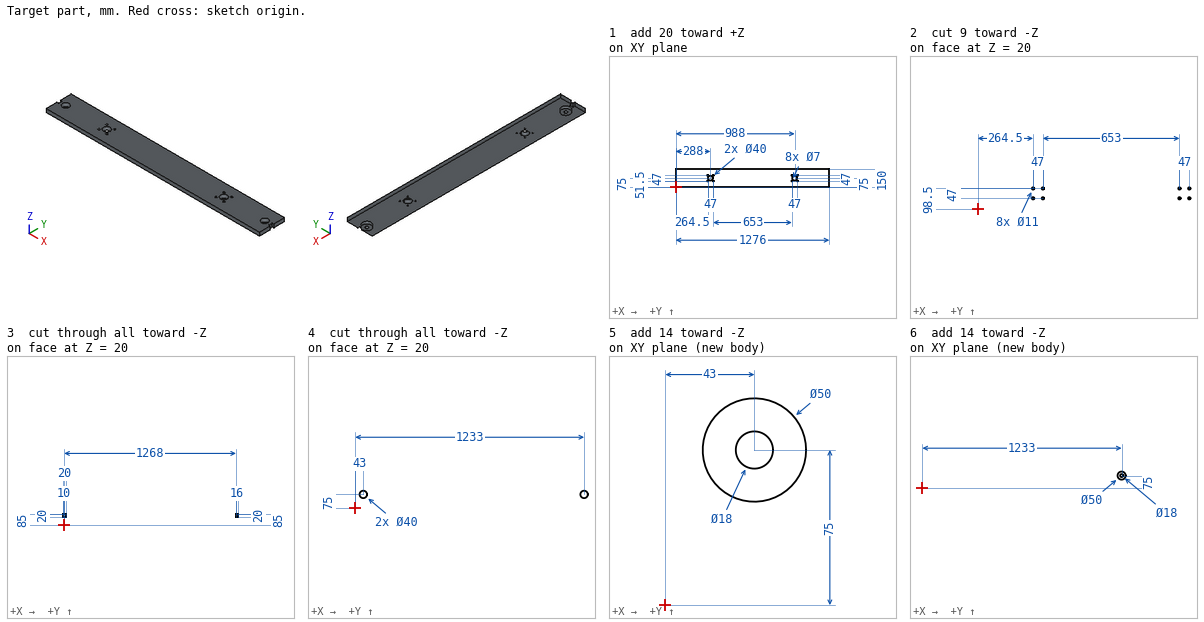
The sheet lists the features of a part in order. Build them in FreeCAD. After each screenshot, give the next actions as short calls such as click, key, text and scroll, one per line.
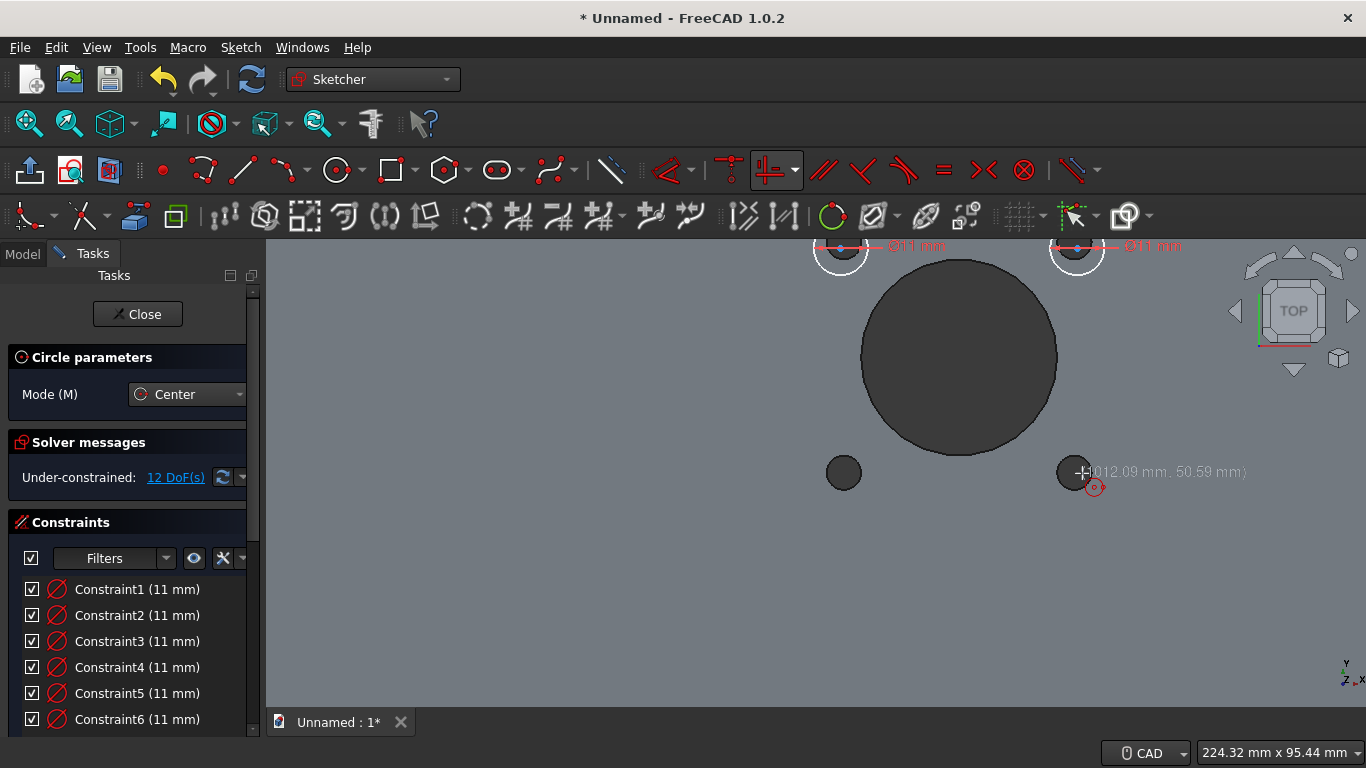
scroll(1082, 473, down, 10)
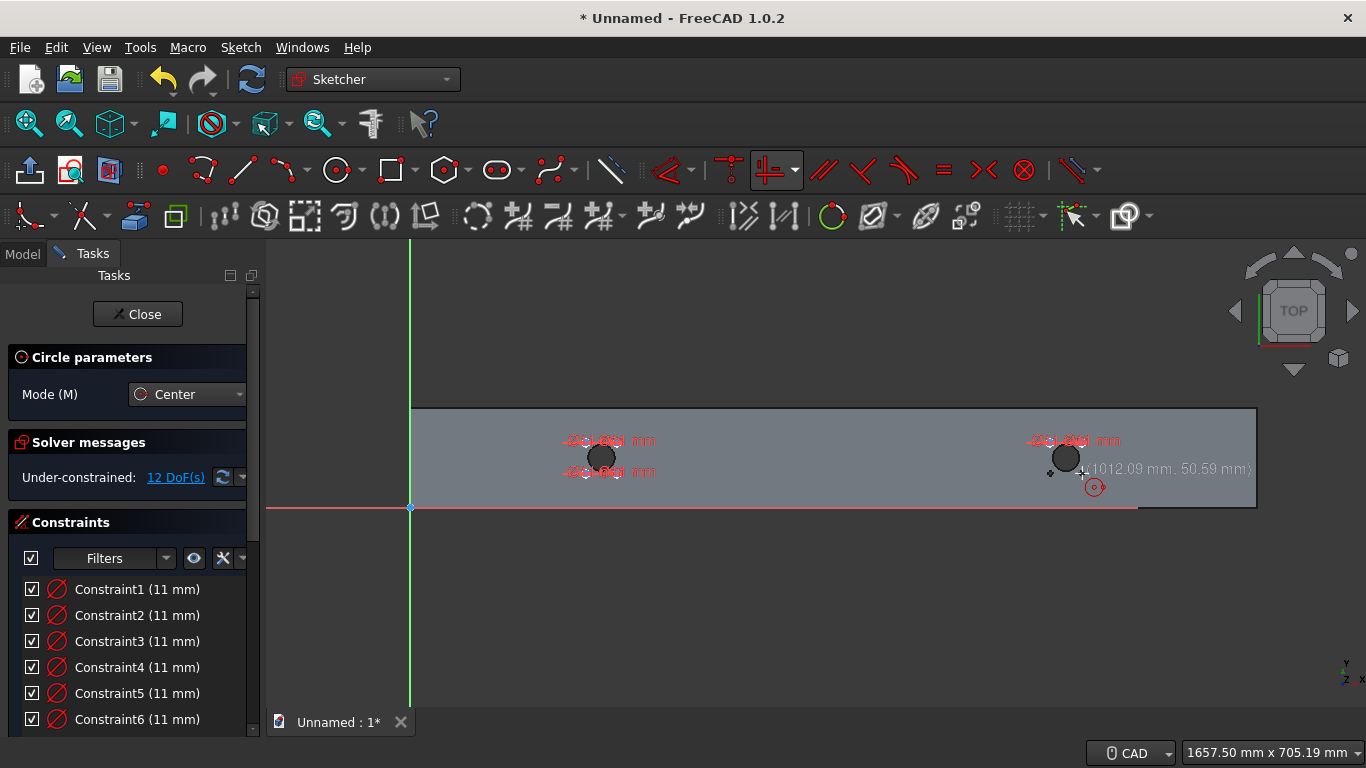
click(1082, 473)
move(1084, 471)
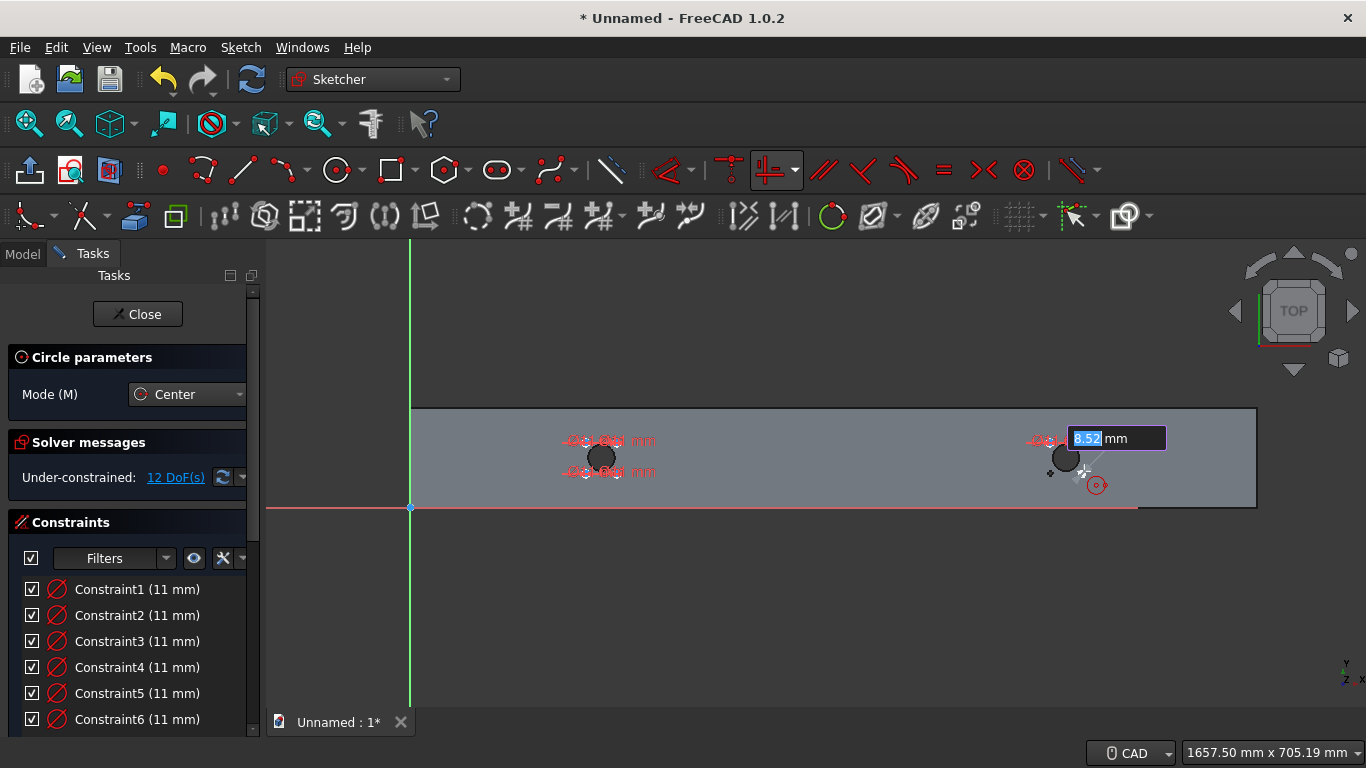
text(11)
key(Return)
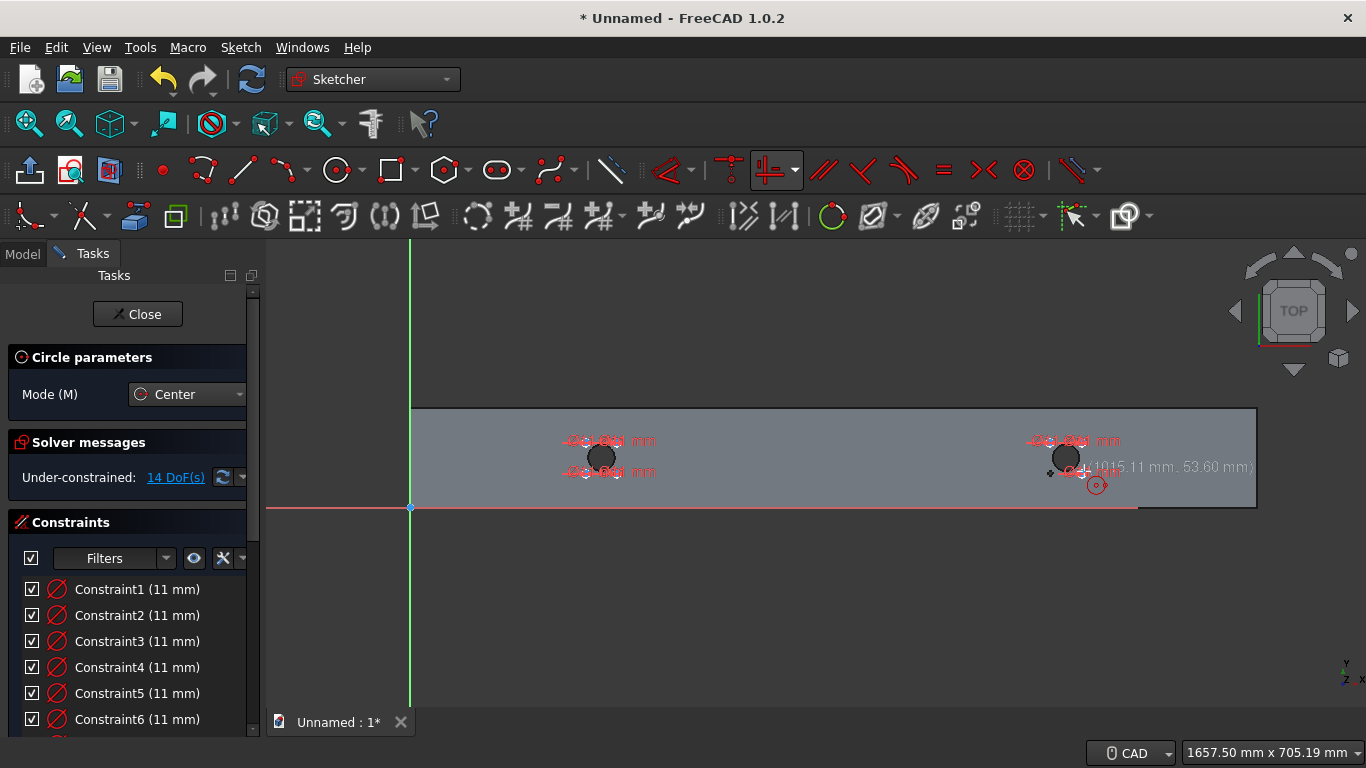
scroll(1050, 473, up, 10)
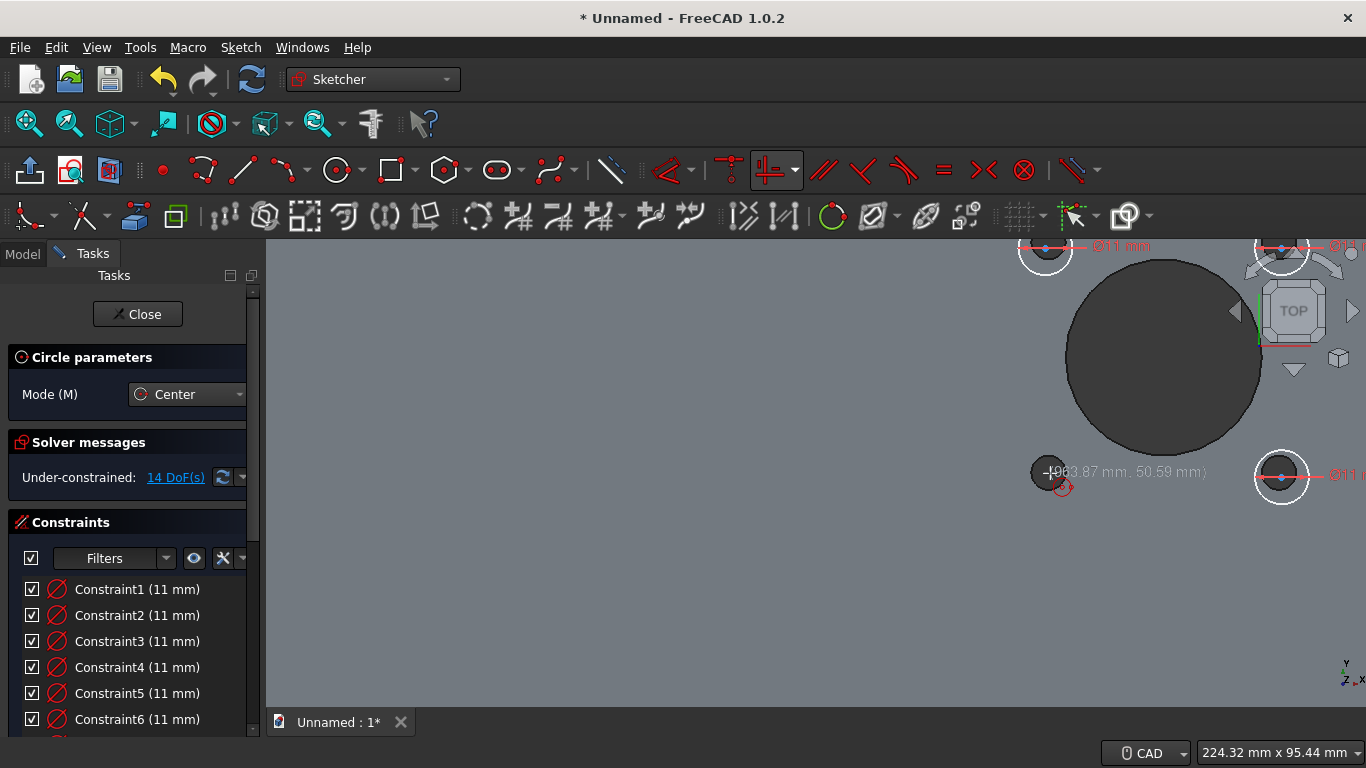
scroll(1050, 473, down, 10)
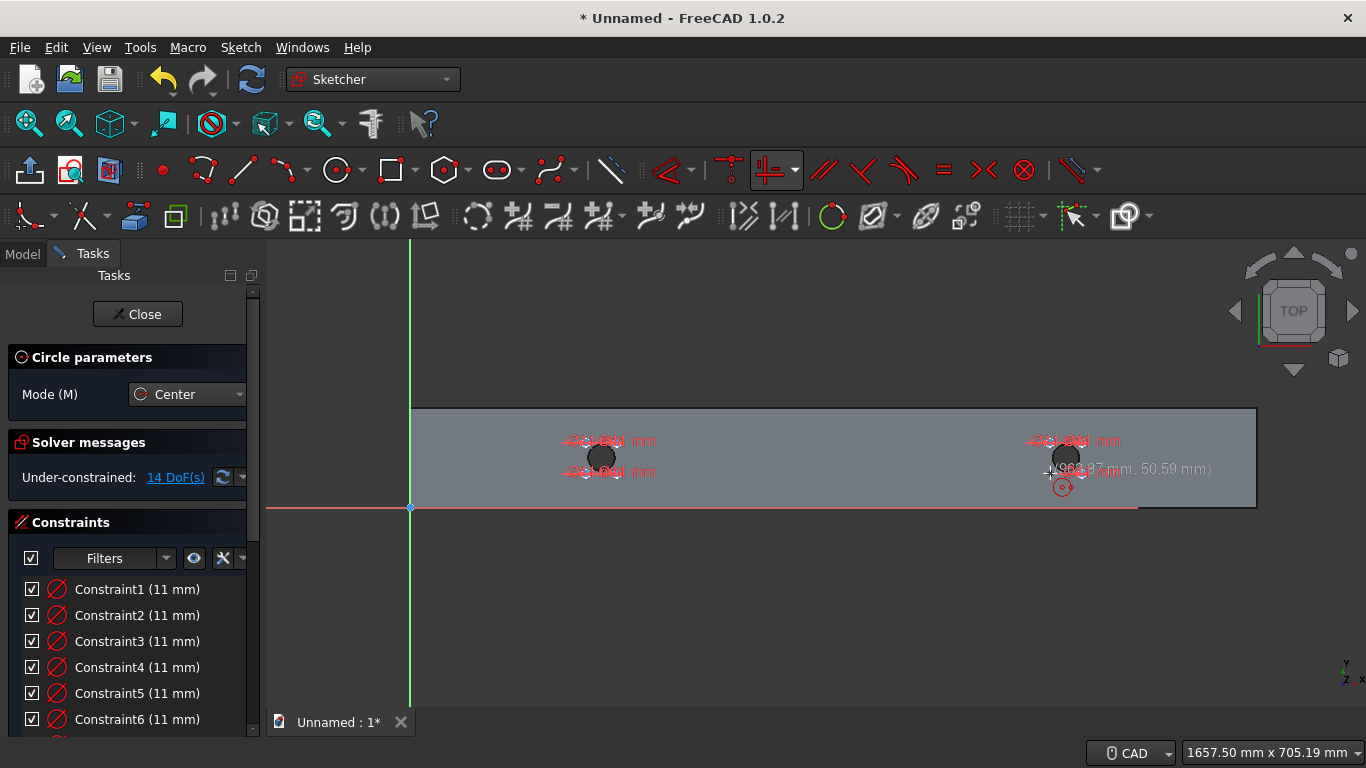
click(1050, 473)
move(1053, 471)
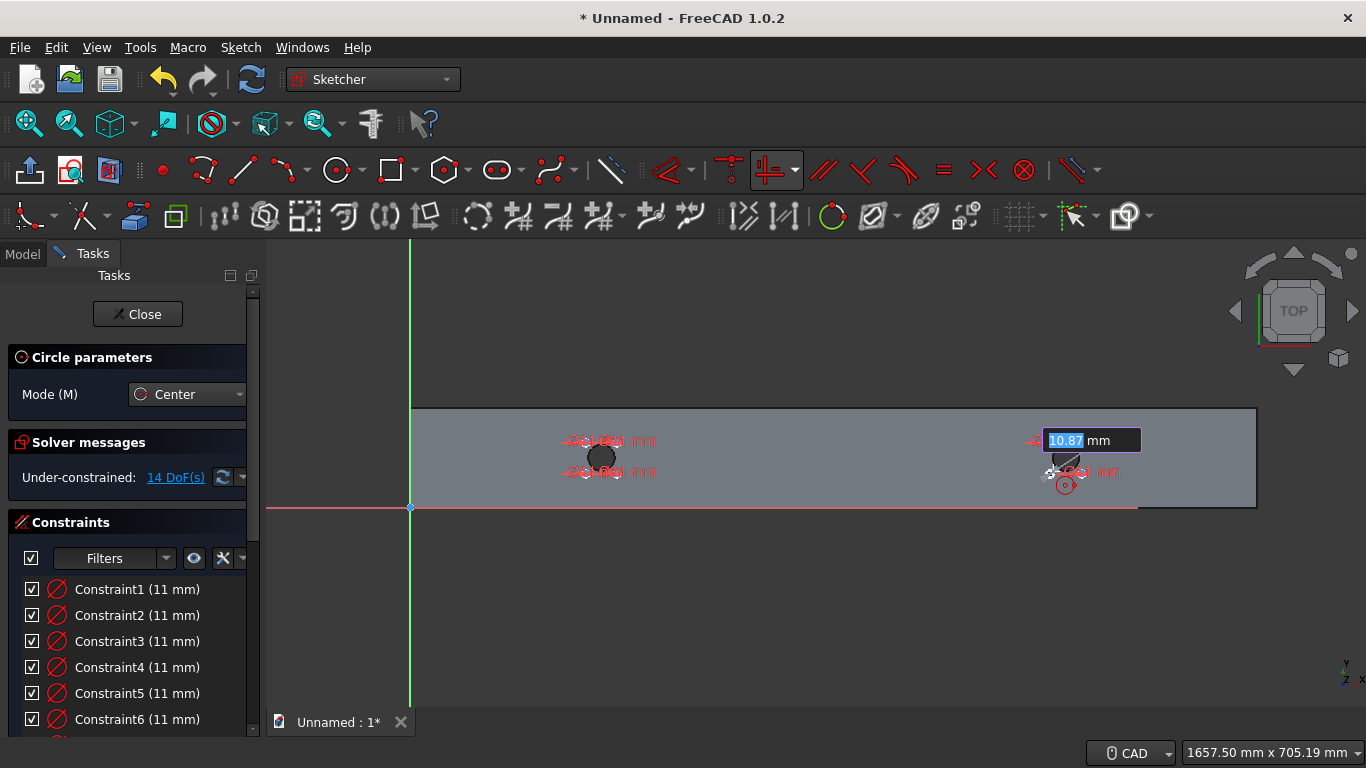
text(11)
key(Return)
key(Escape)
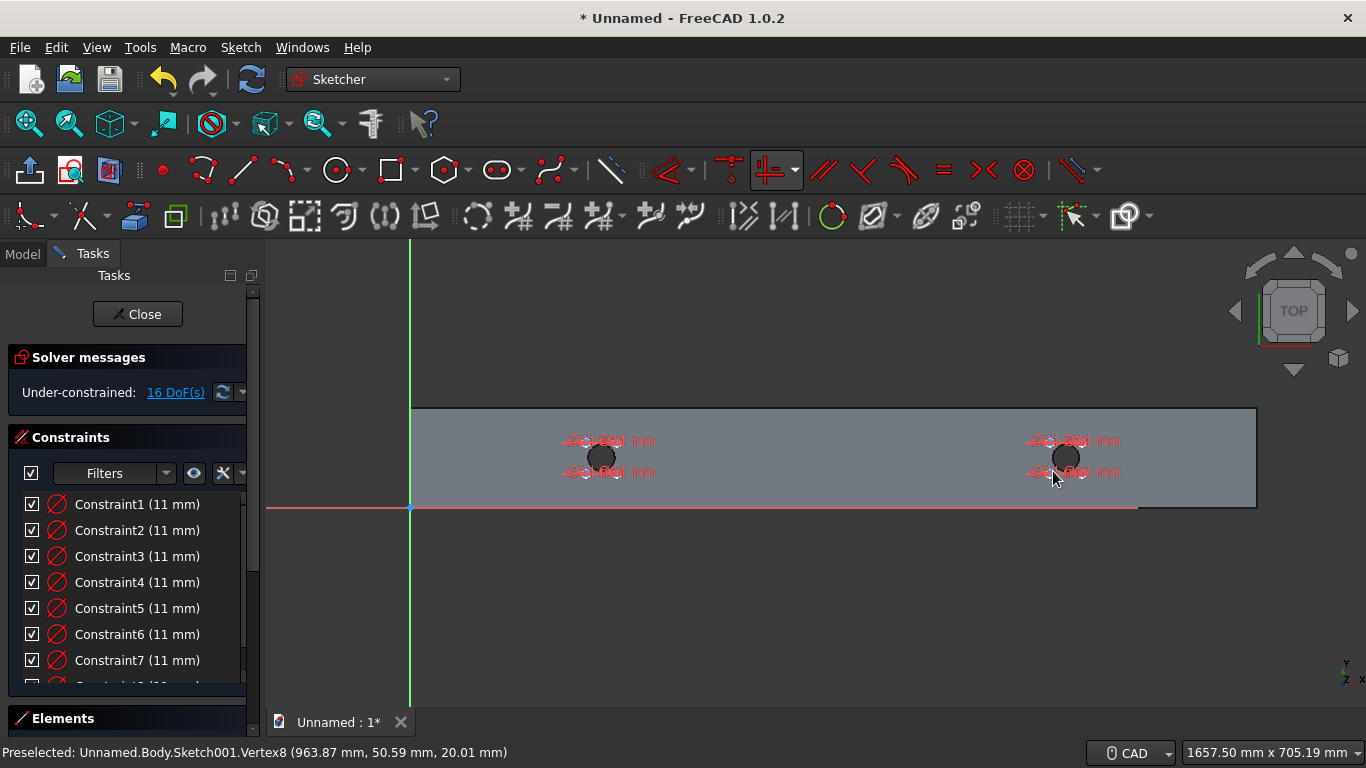
click(586, 443)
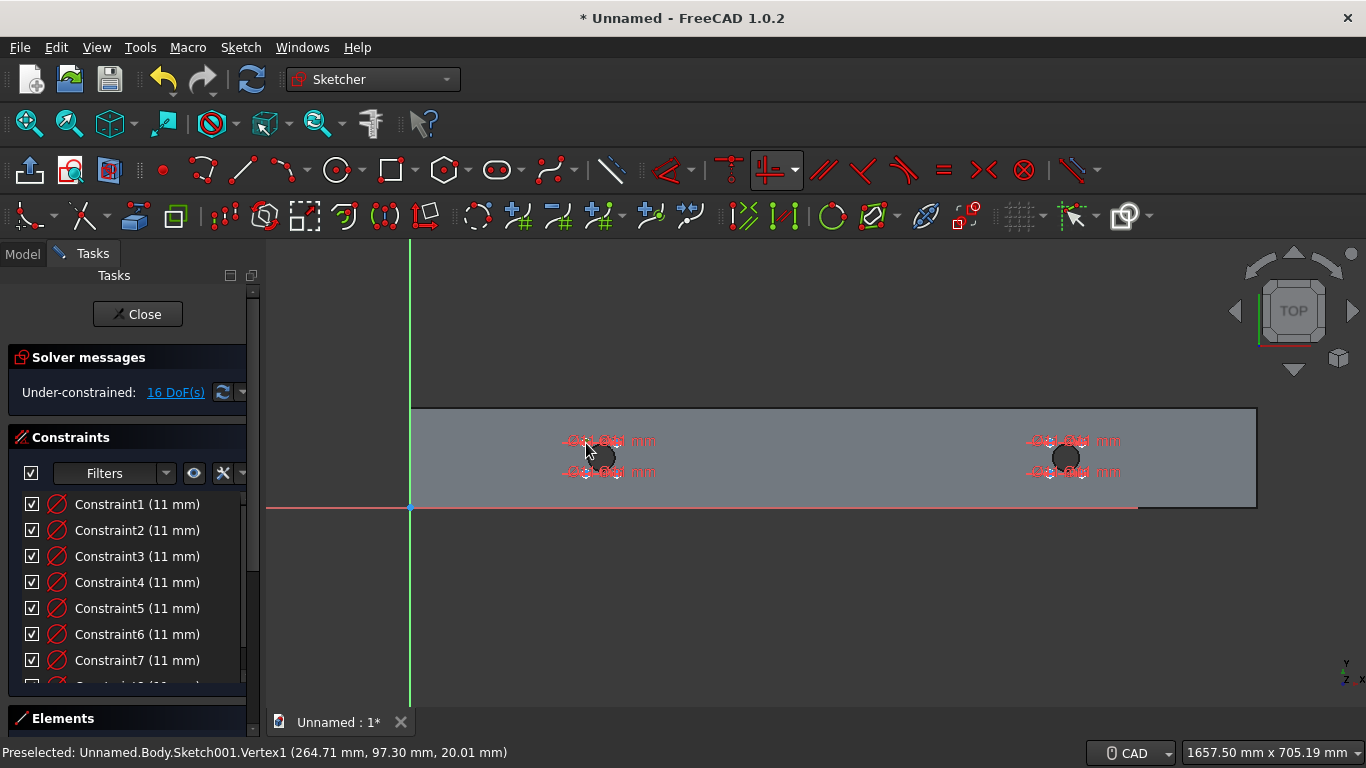
click(617, 443)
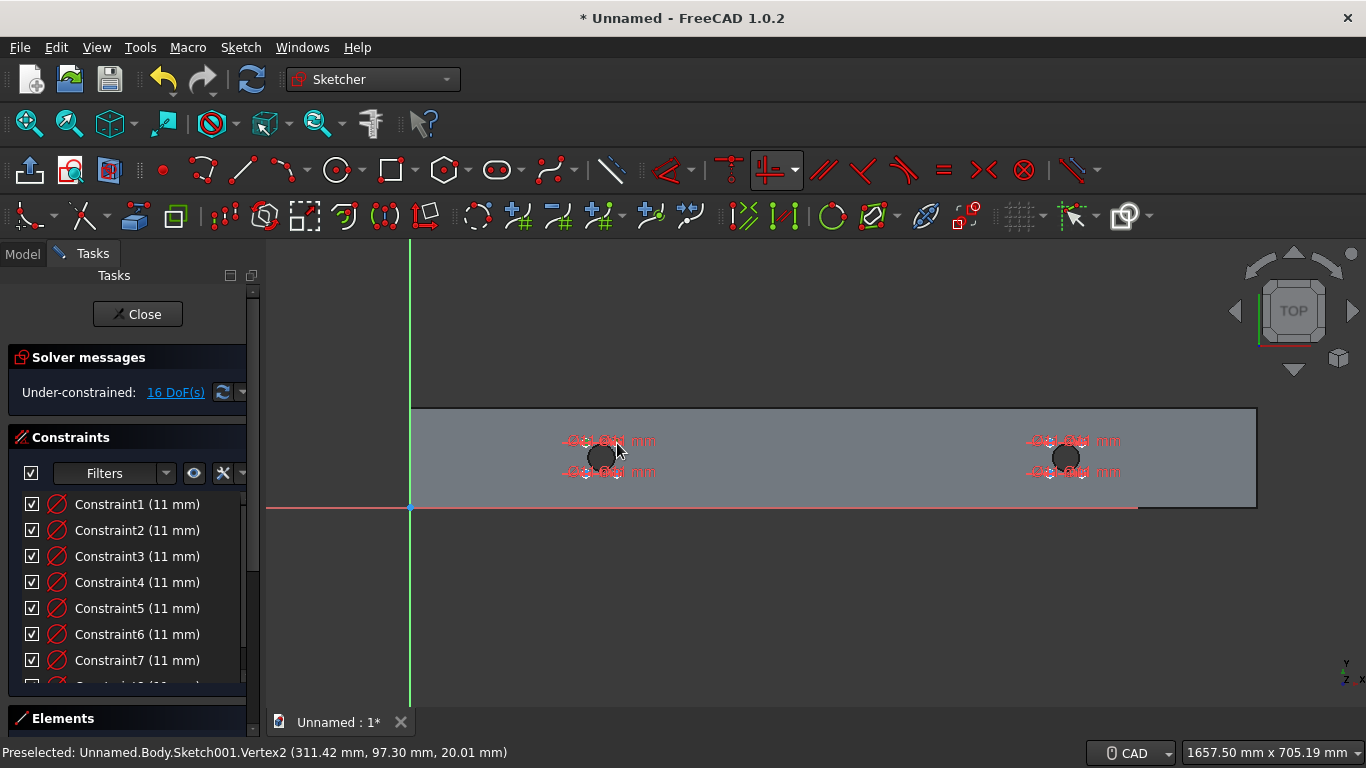
click(798, 170)